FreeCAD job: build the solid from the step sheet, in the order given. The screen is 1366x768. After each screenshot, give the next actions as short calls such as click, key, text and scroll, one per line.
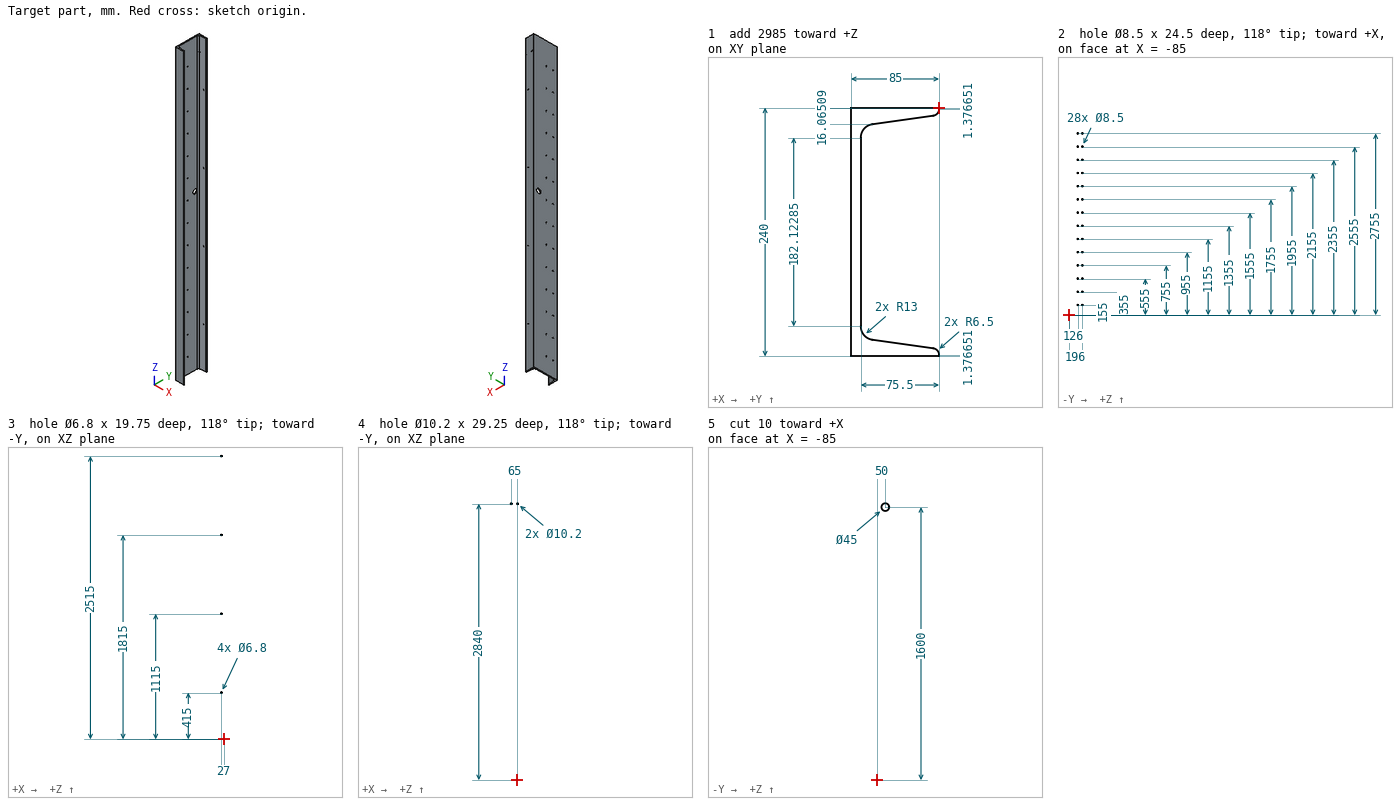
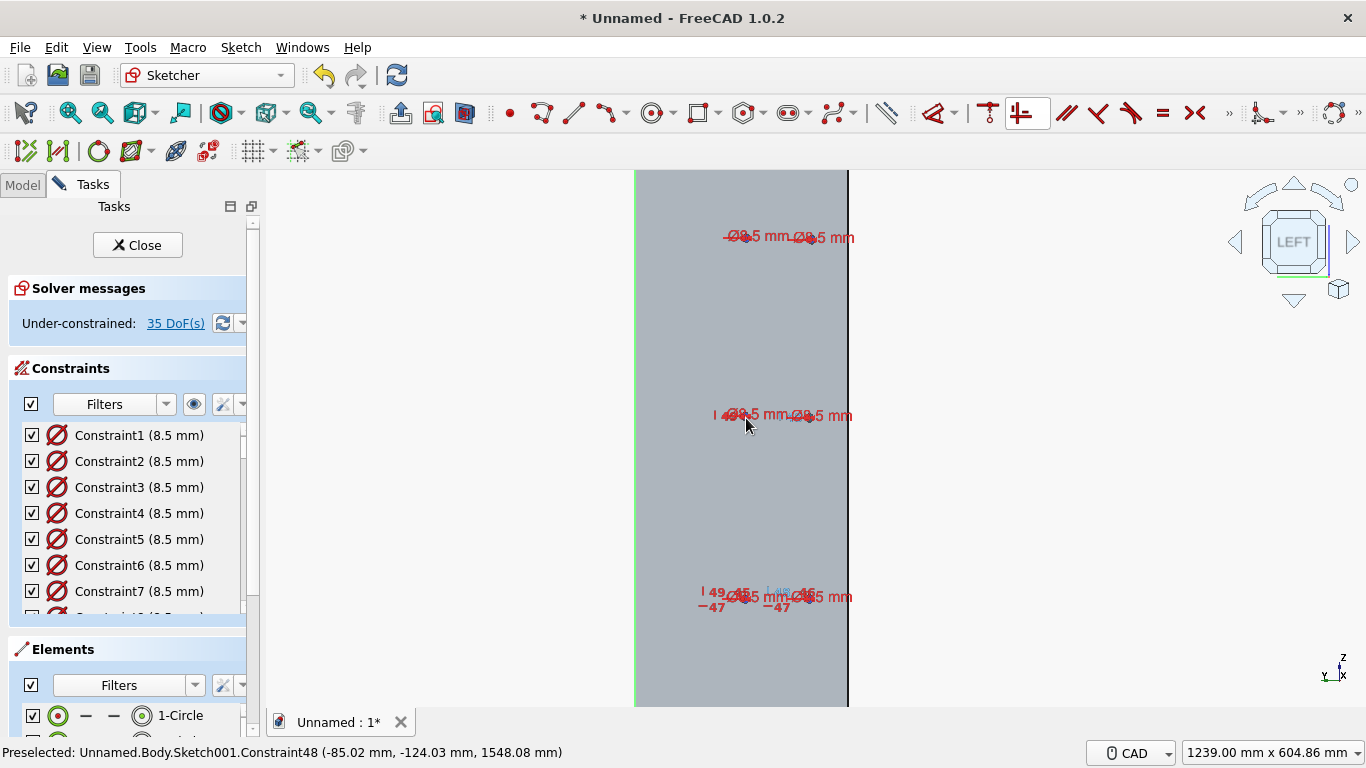
click(745, 416)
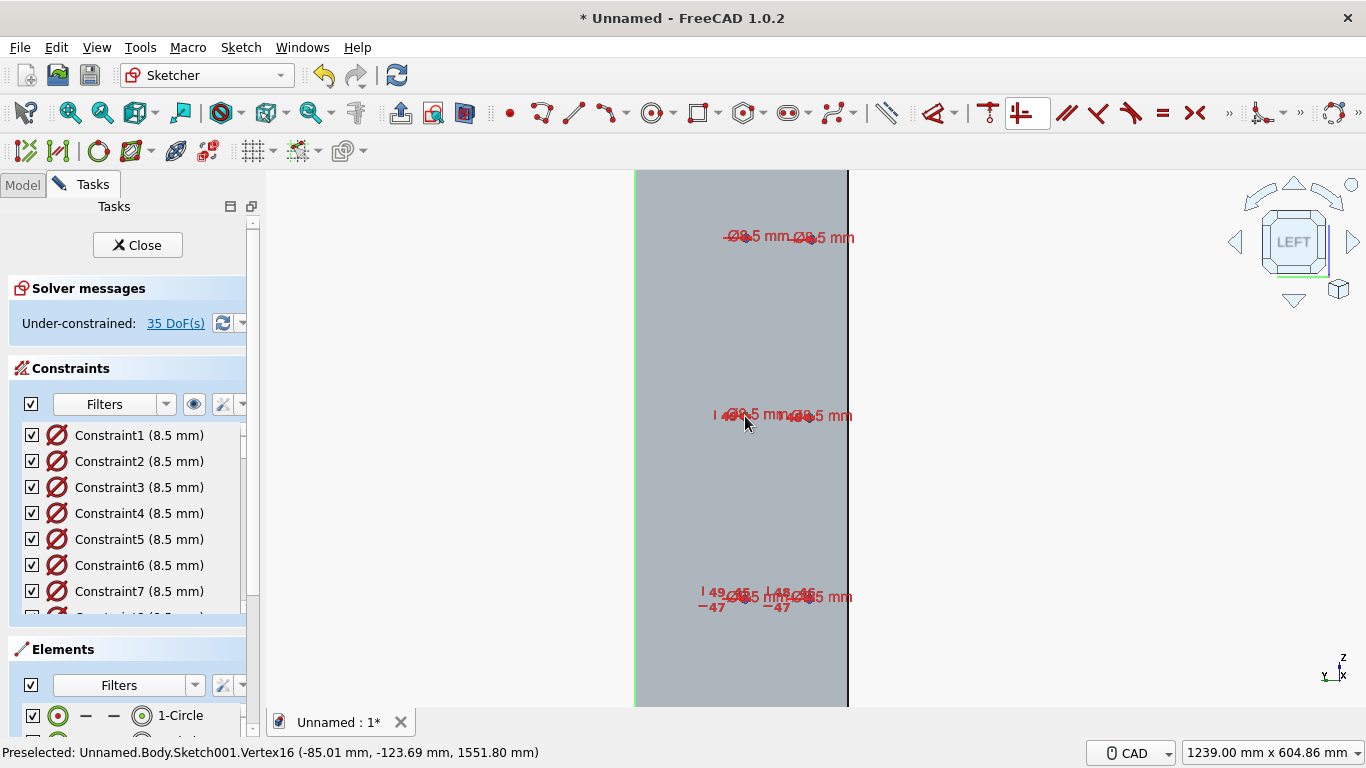
key(h)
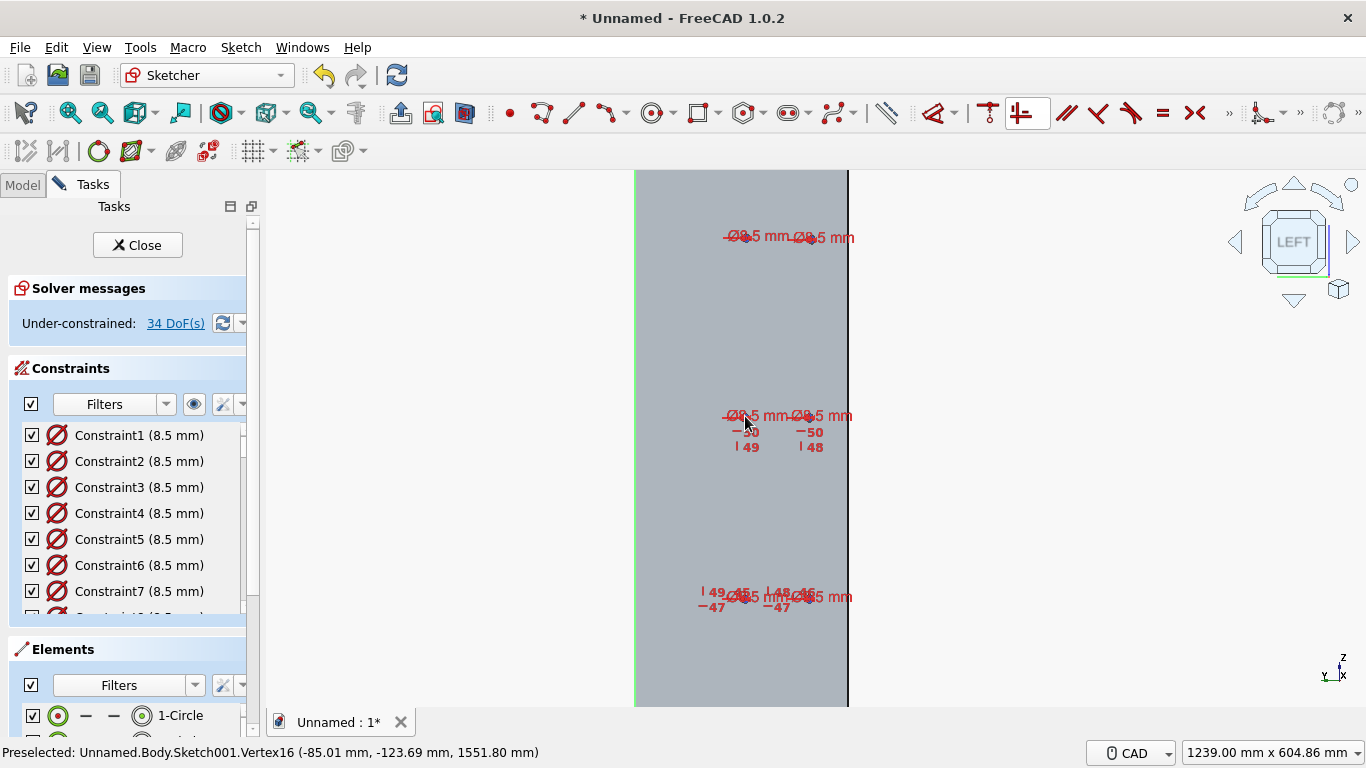
scroll(751, 418, down, 10)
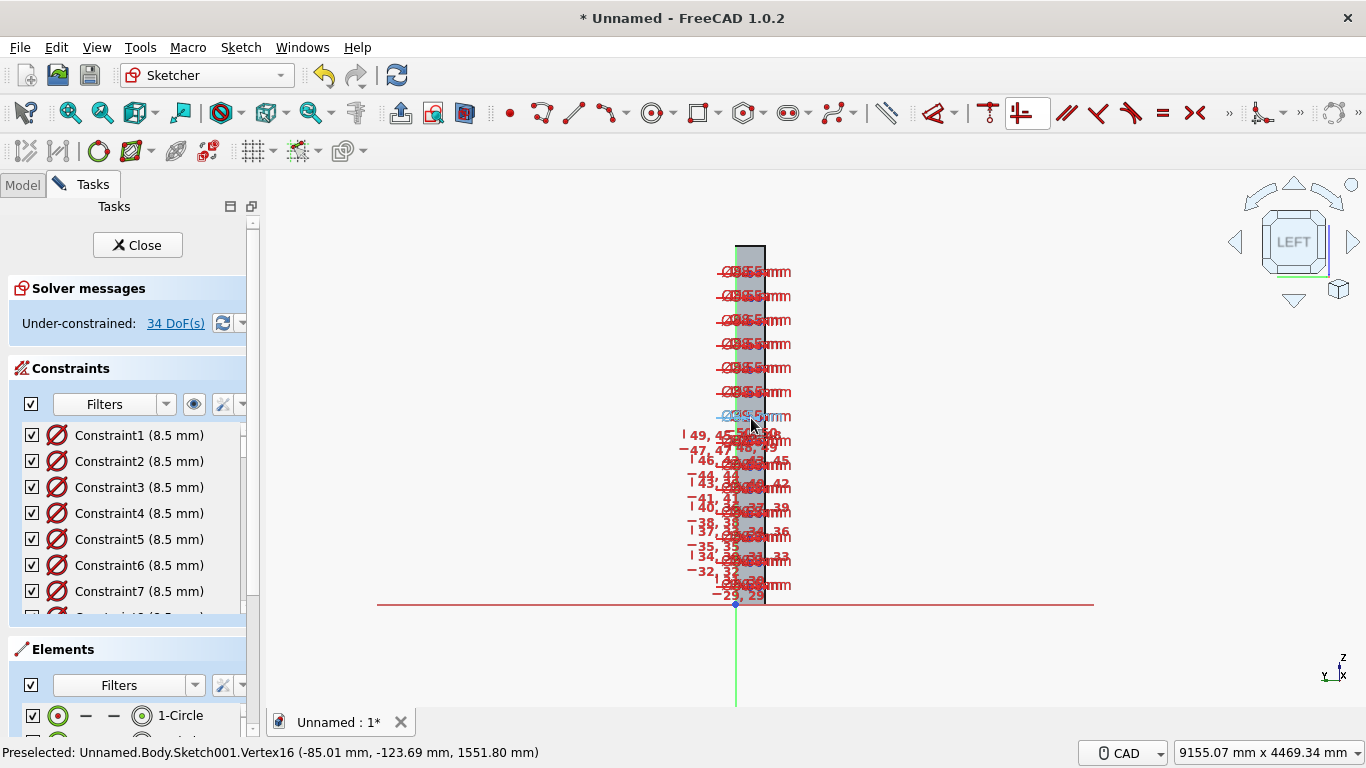
scroll(759, 418, up, 2)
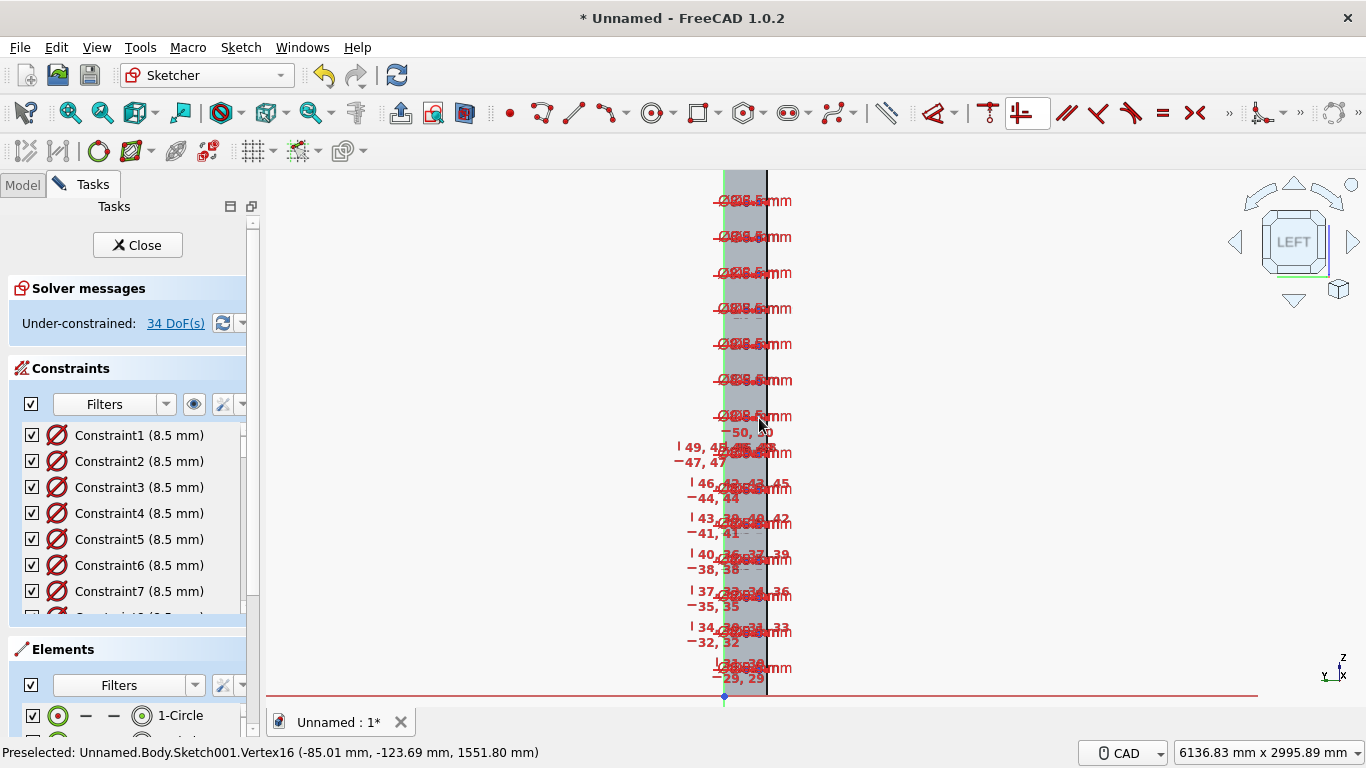
click(759, 418)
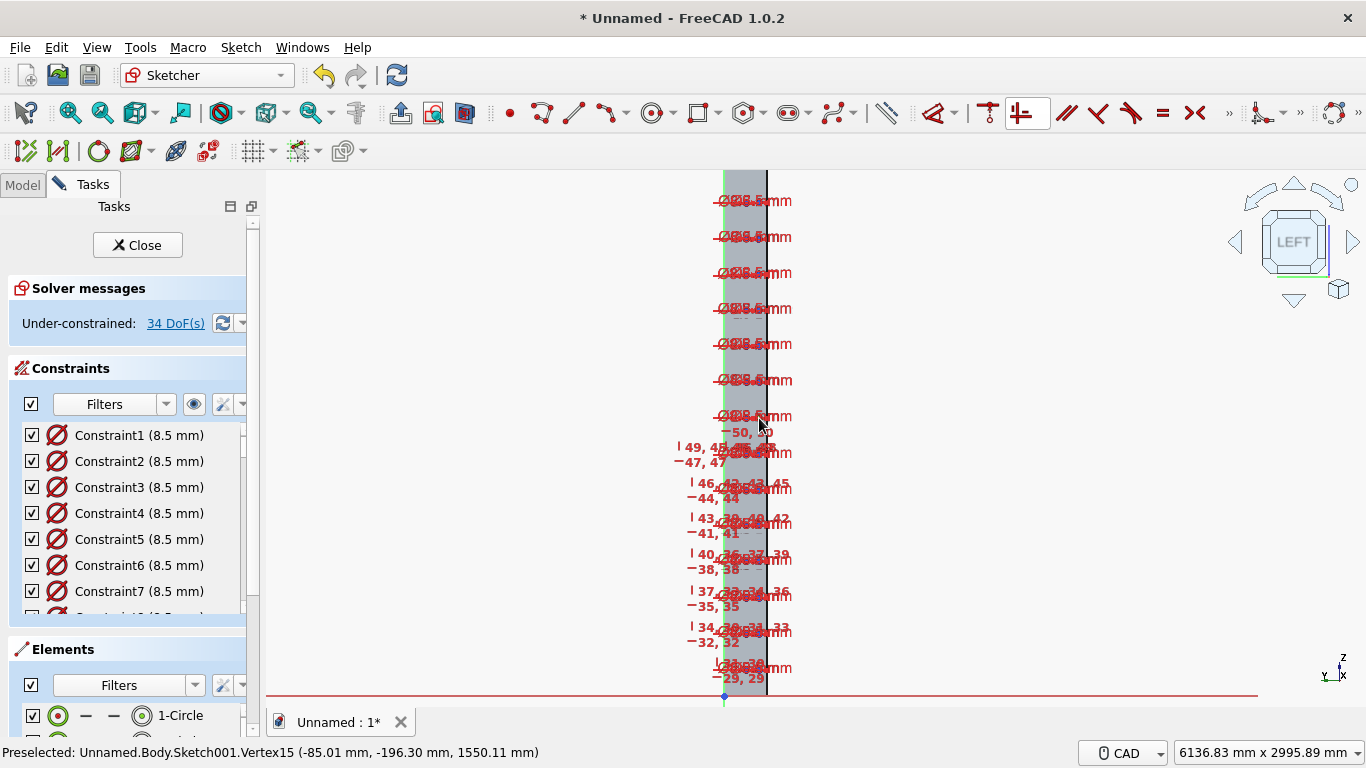
click(760, 382)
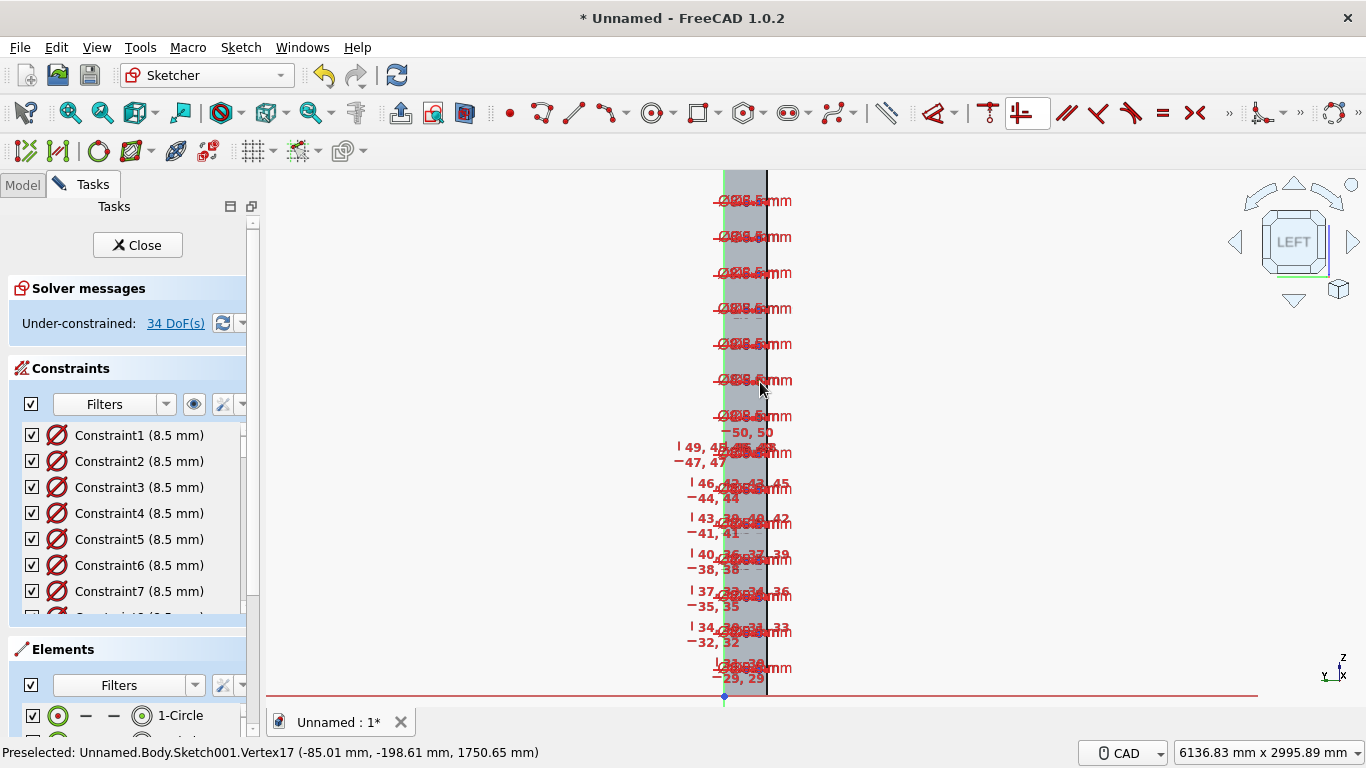
click(1044, 114)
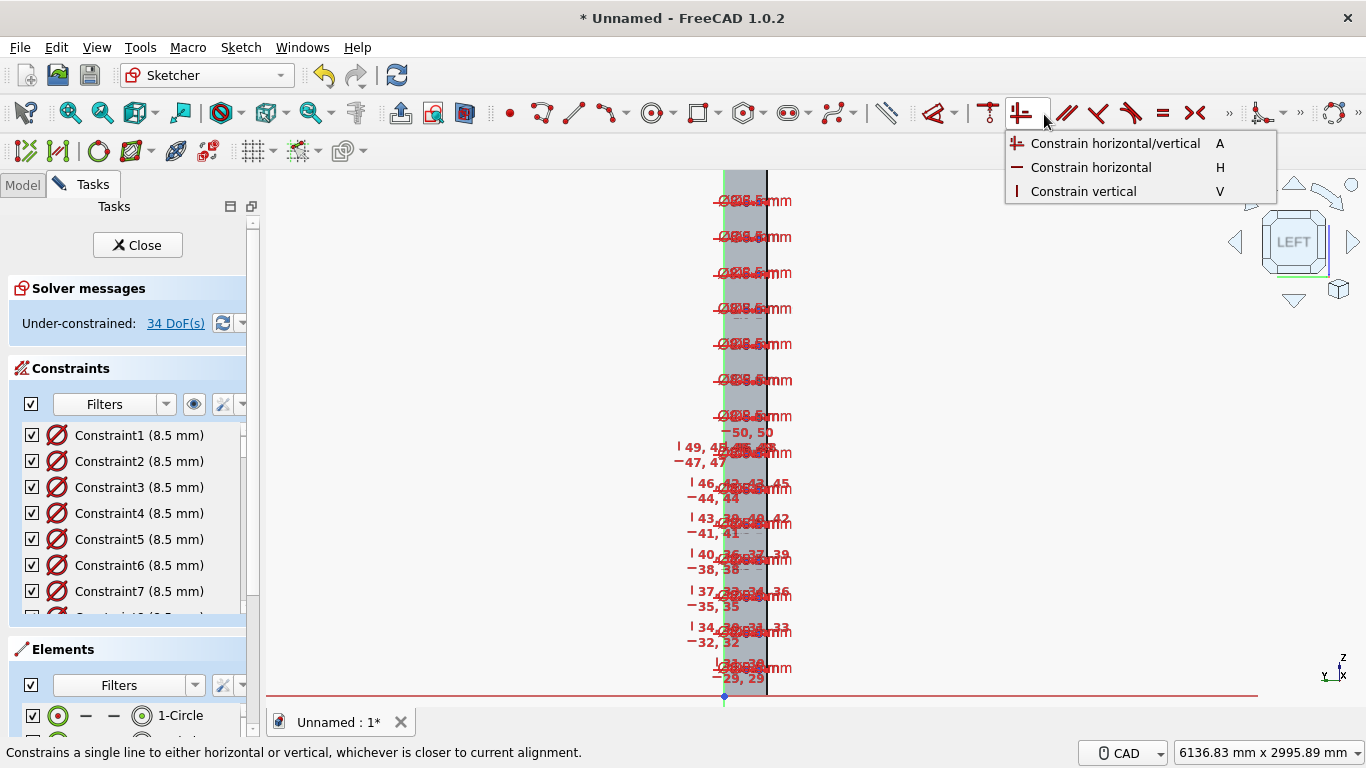
click(1141, 191)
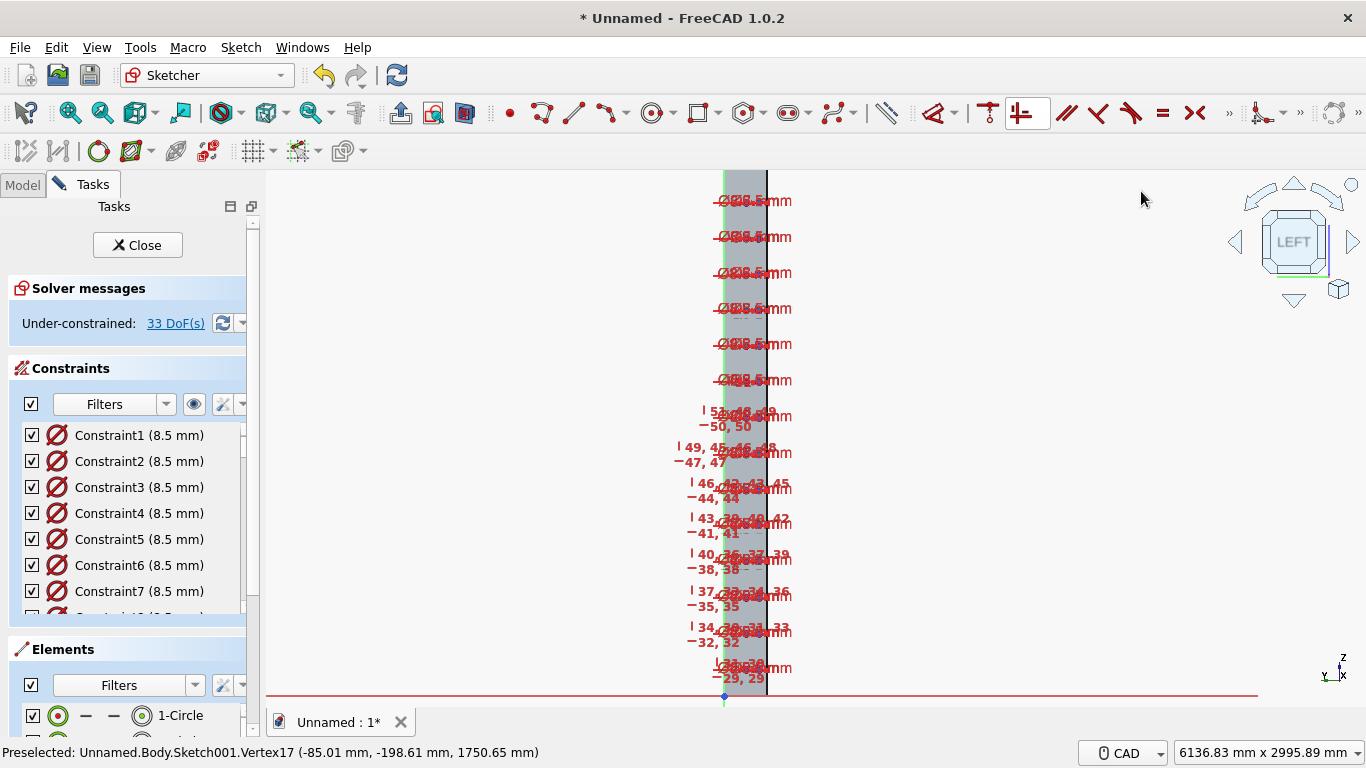
click(746, 418)